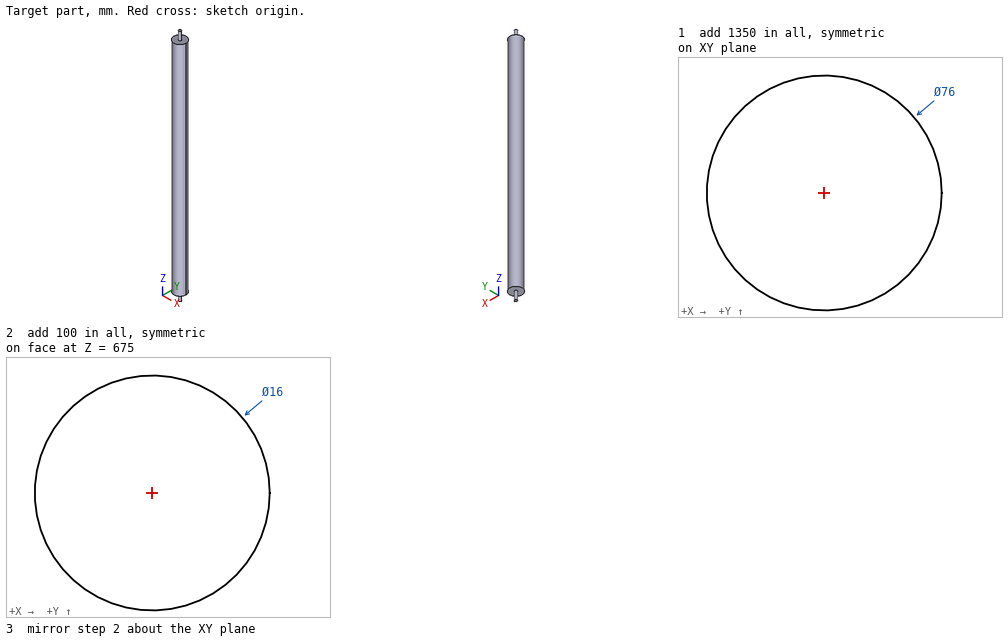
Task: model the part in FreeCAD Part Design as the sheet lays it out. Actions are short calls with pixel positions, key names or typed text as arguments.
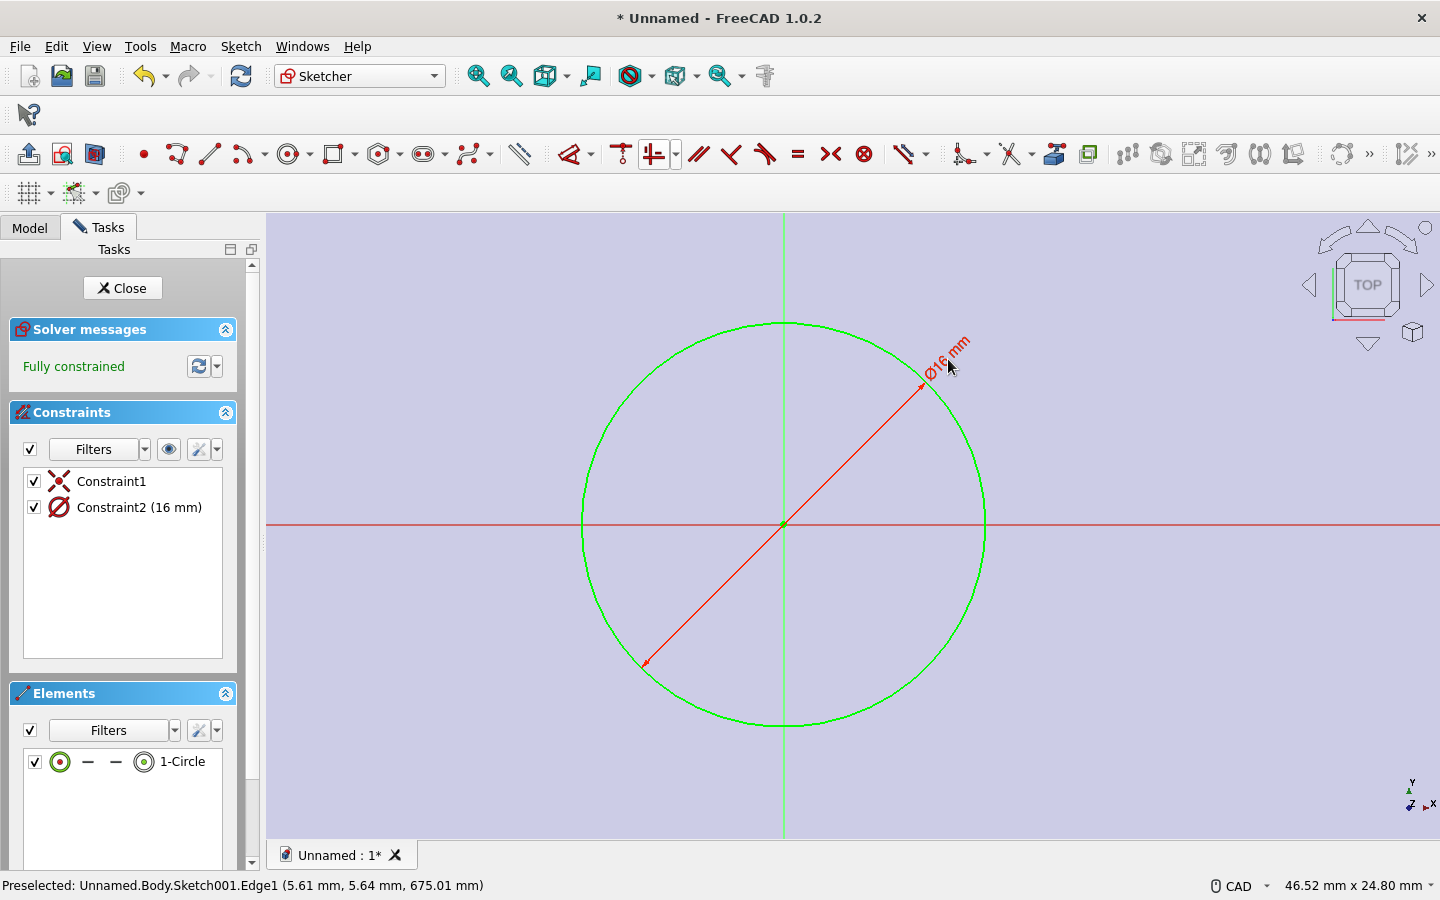
click(123, 288)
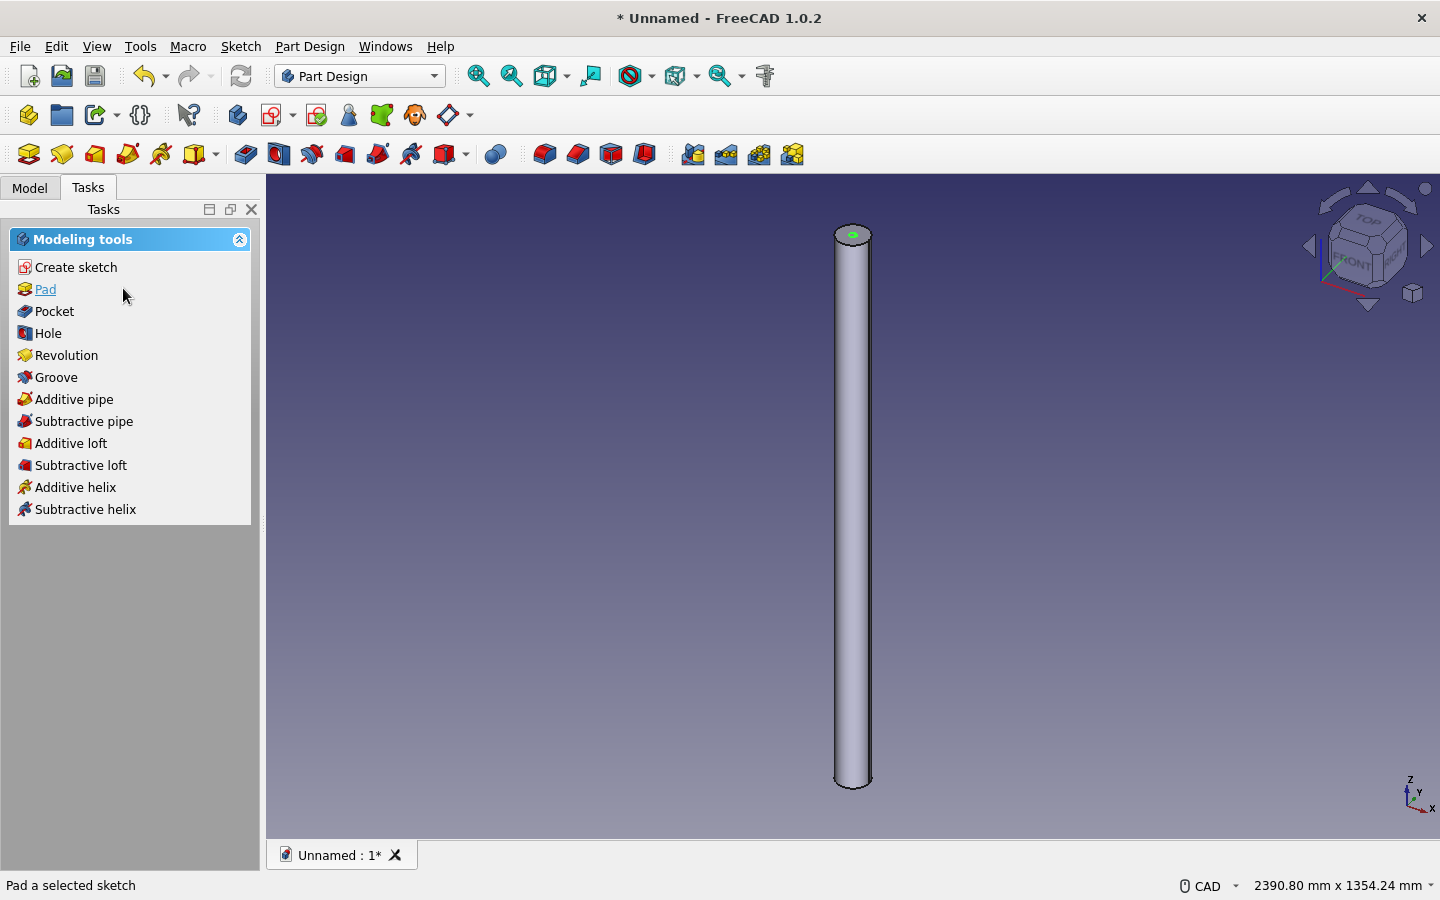
click(29, 154)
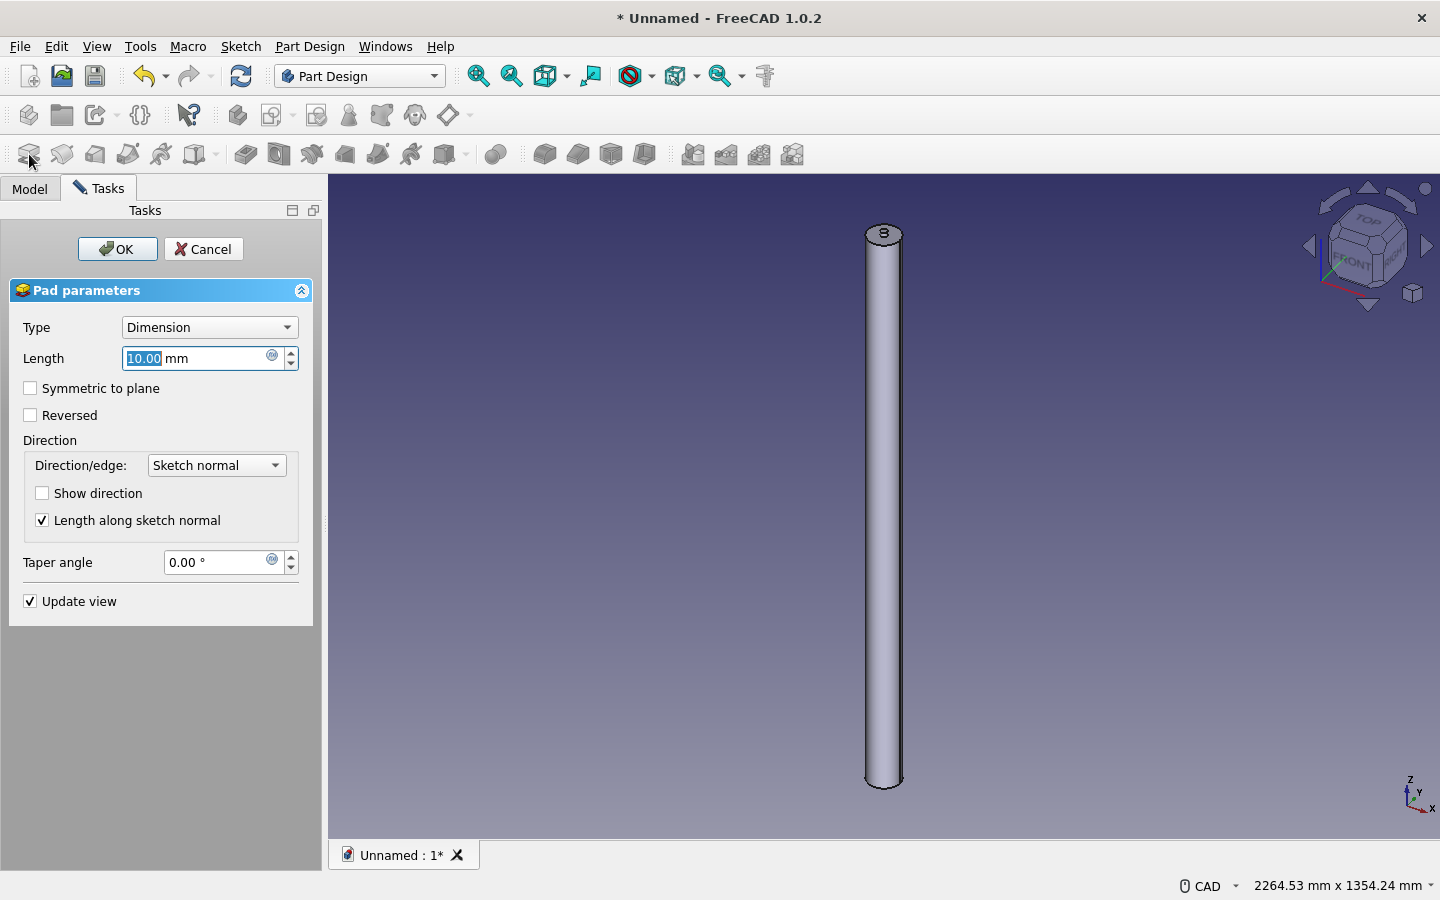
text(100)
key(Tab)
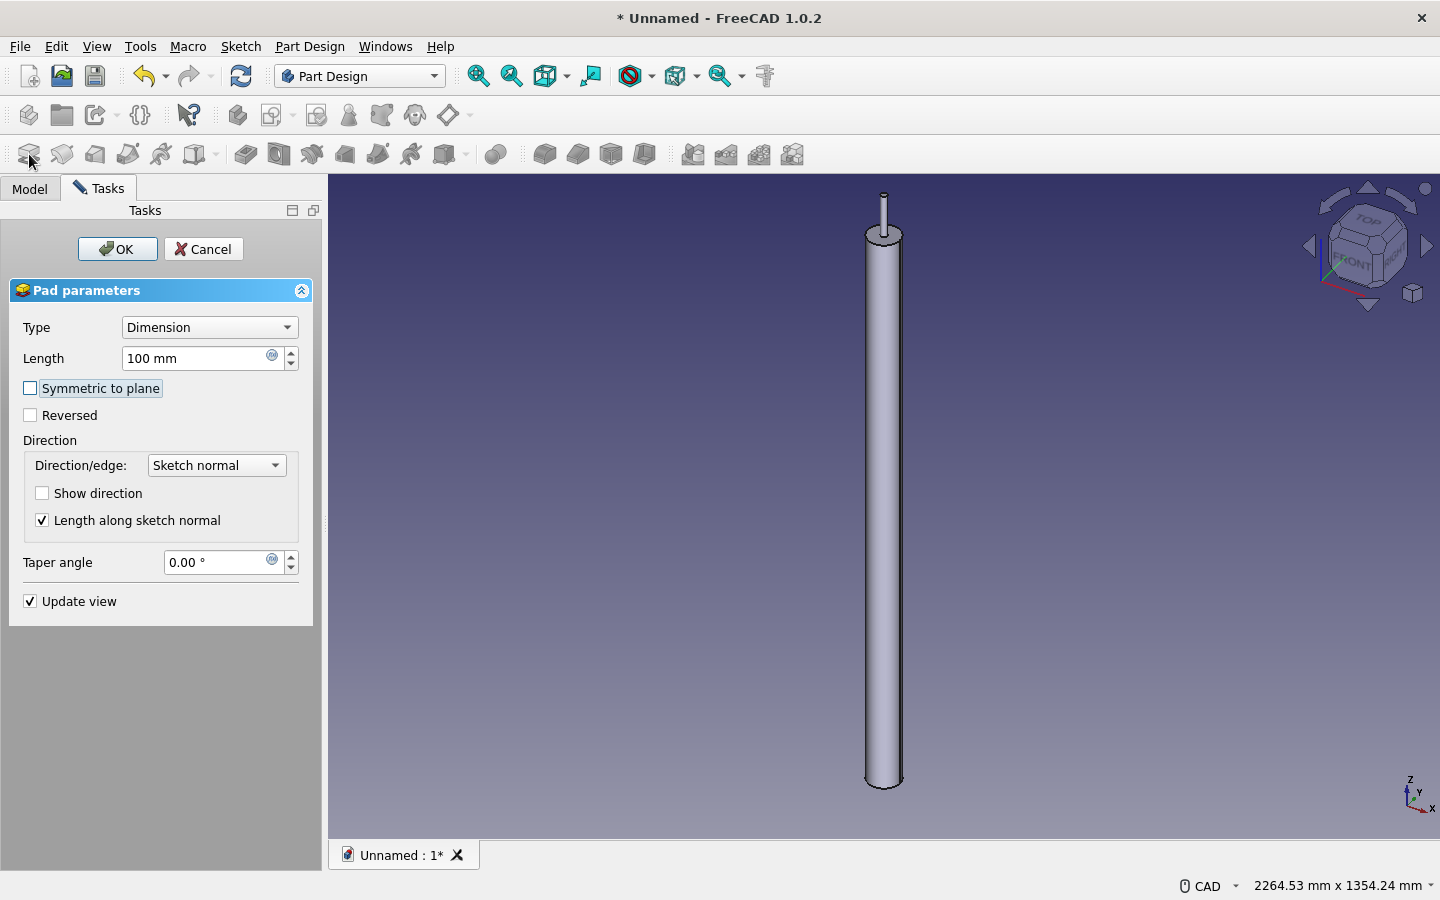
click(31, 388)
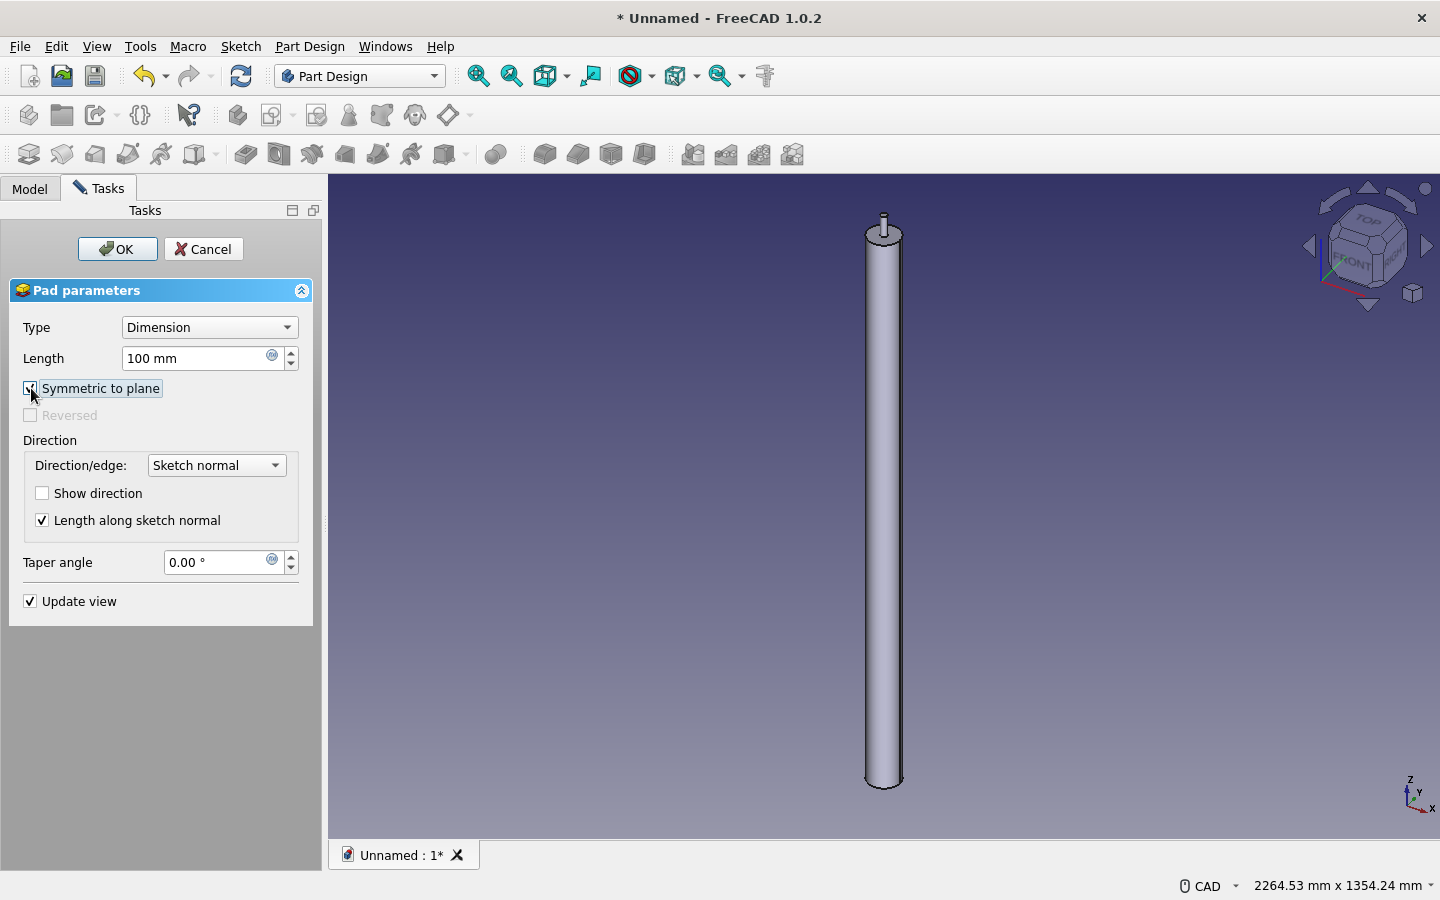
click(118, 249)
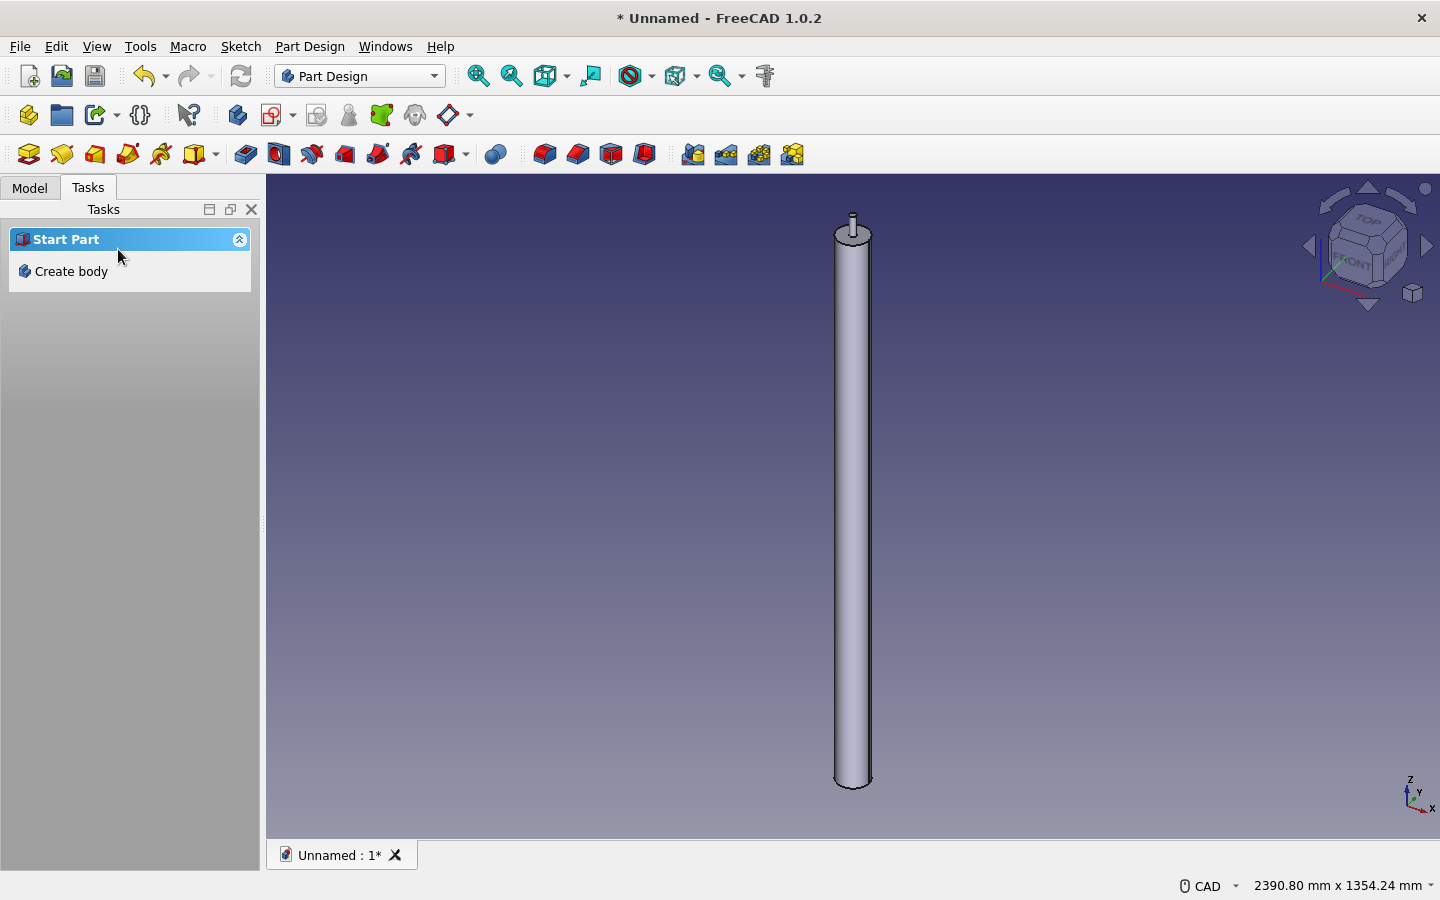
click(30, 188)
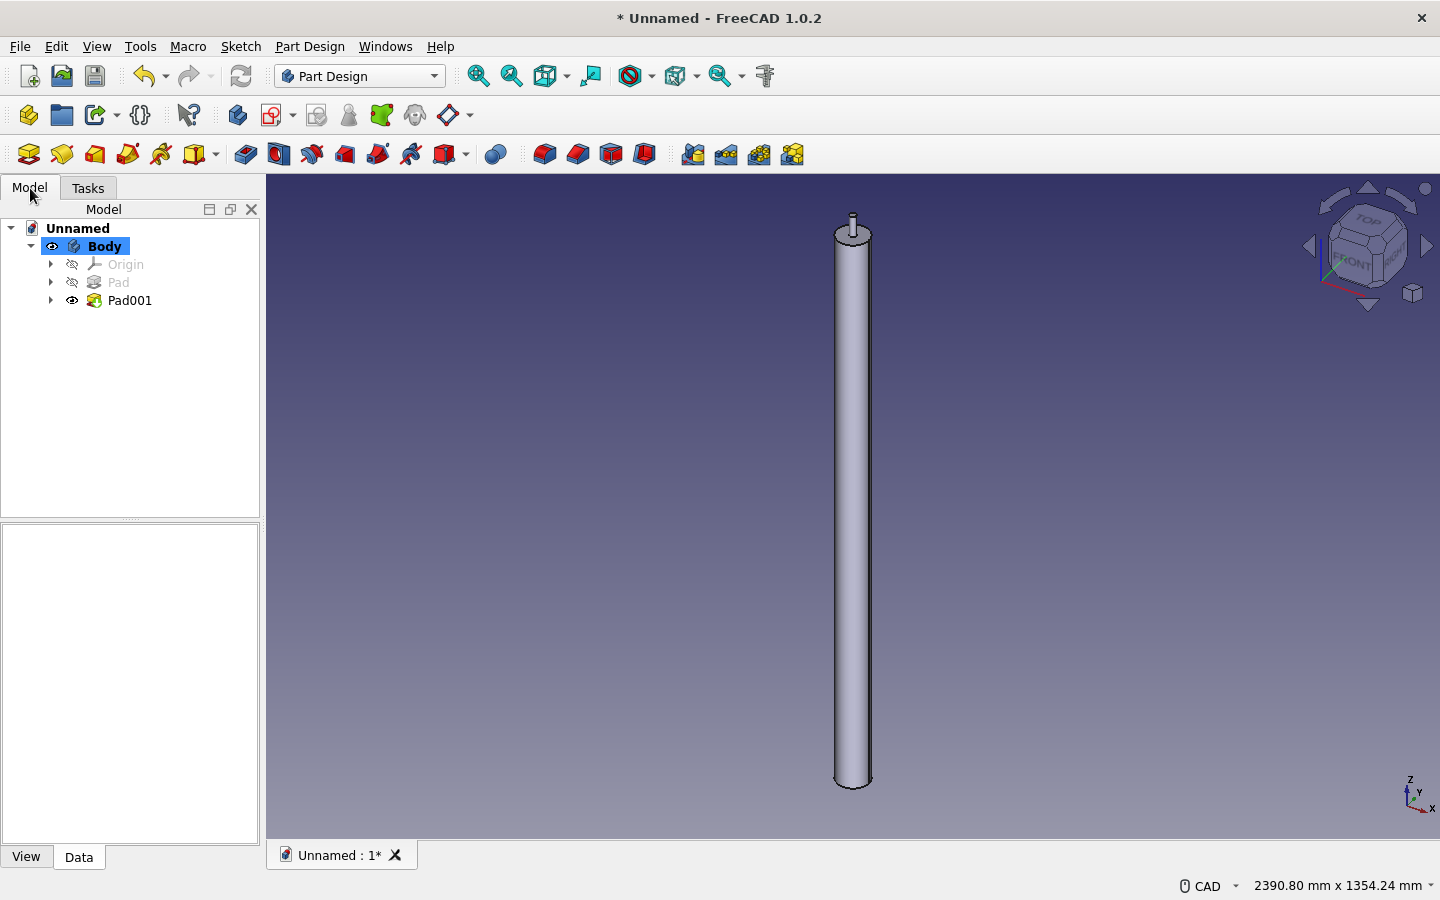
click(117, 300)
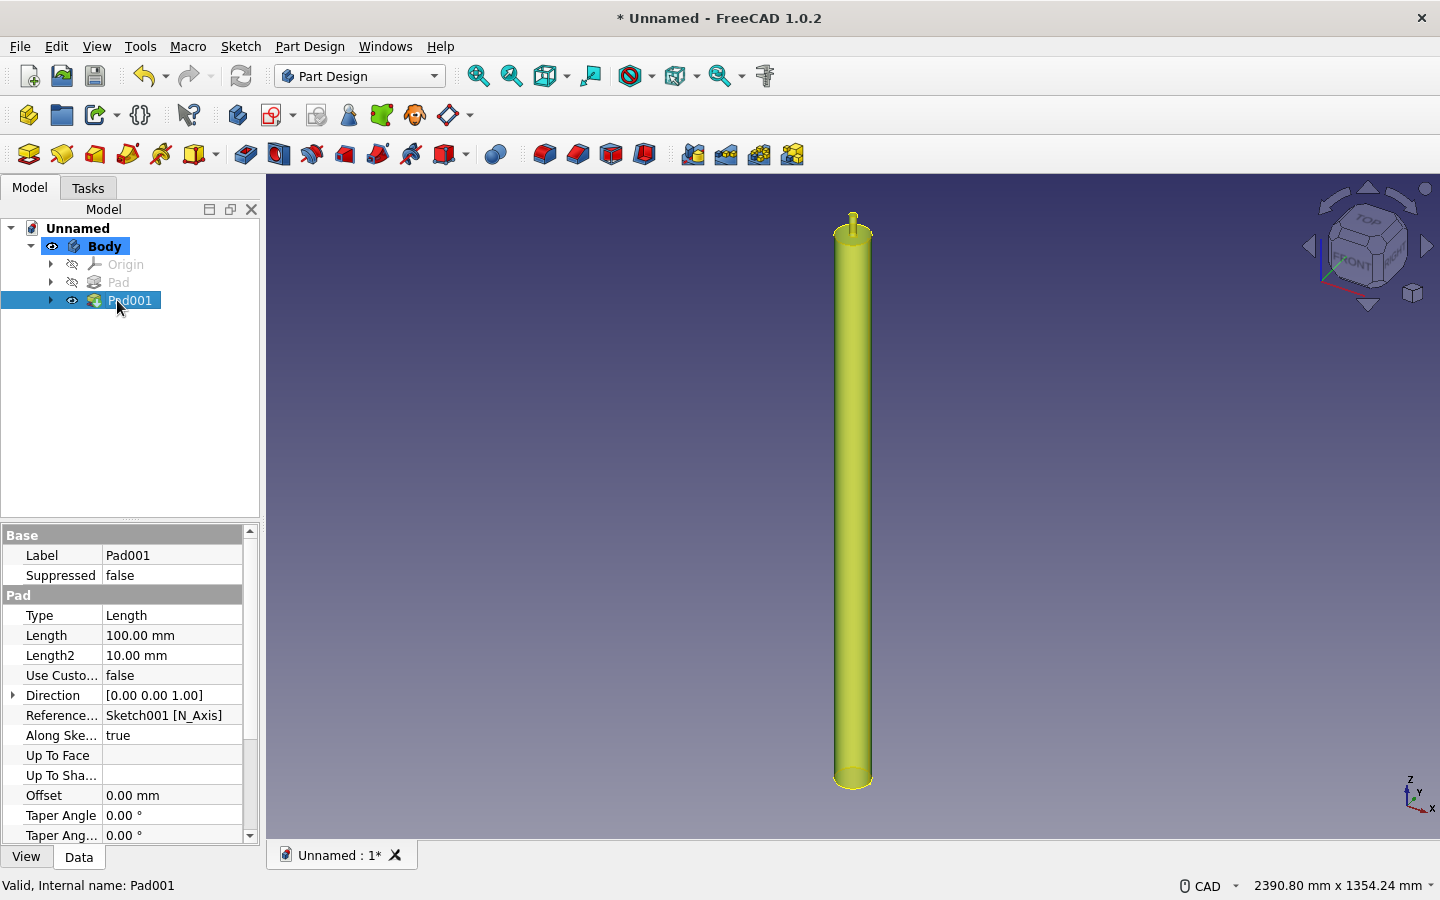
click(693, 154)